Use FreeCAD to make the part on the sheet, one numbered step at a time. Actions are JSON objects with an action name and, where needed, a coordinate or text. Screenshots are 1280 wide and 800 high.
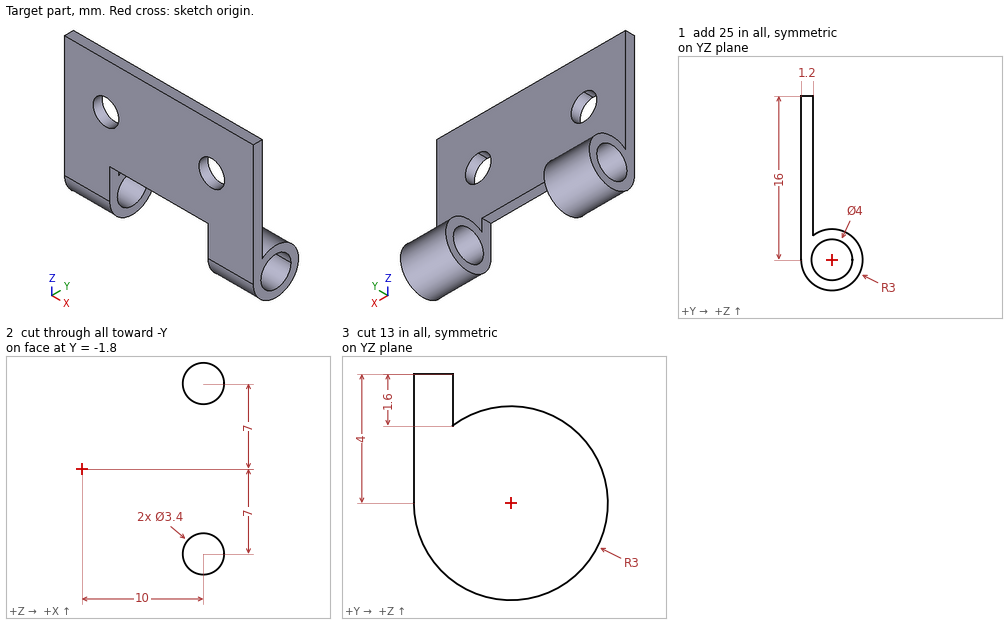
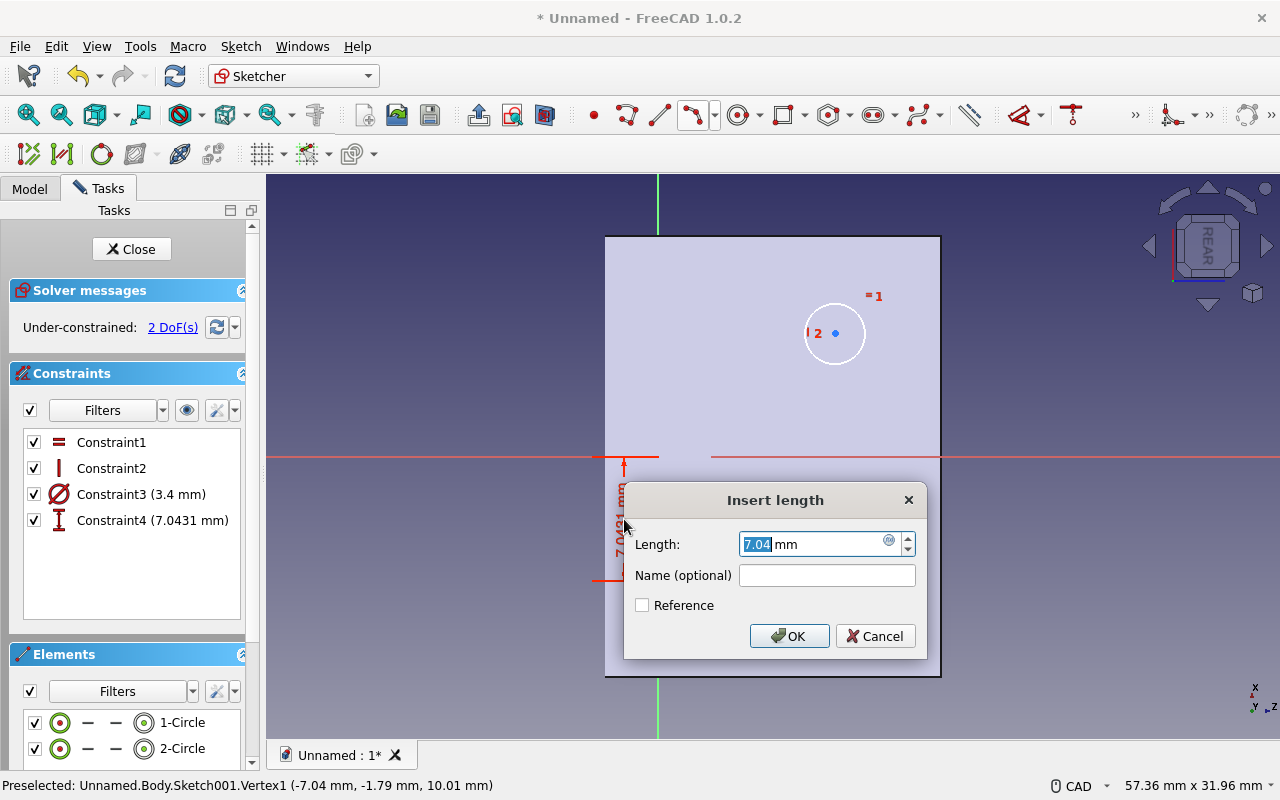
{"action": "type", "text": "7"}
{"action": "key", "text": "Return"}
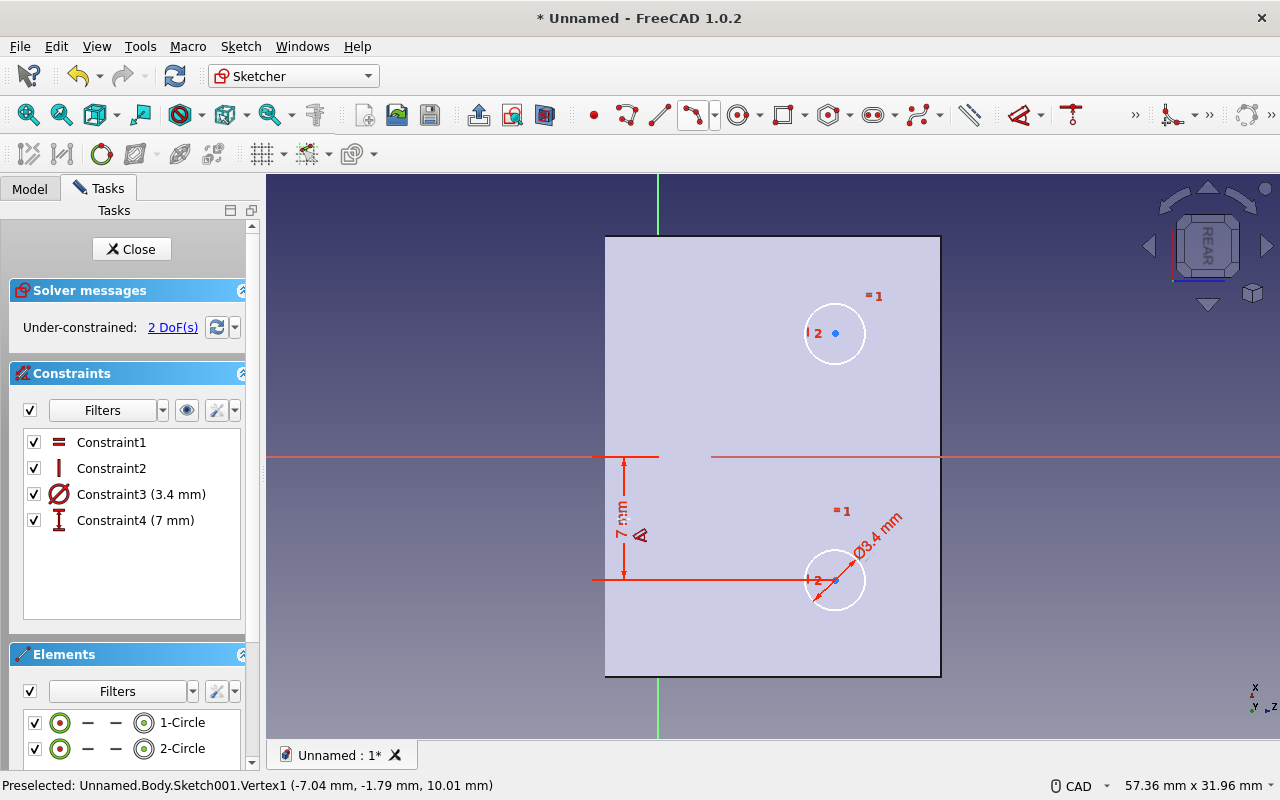
{"action": "left_click", "coordinate": [835, 334]}
{"action": "left_click", "coordinate": [624, 395]}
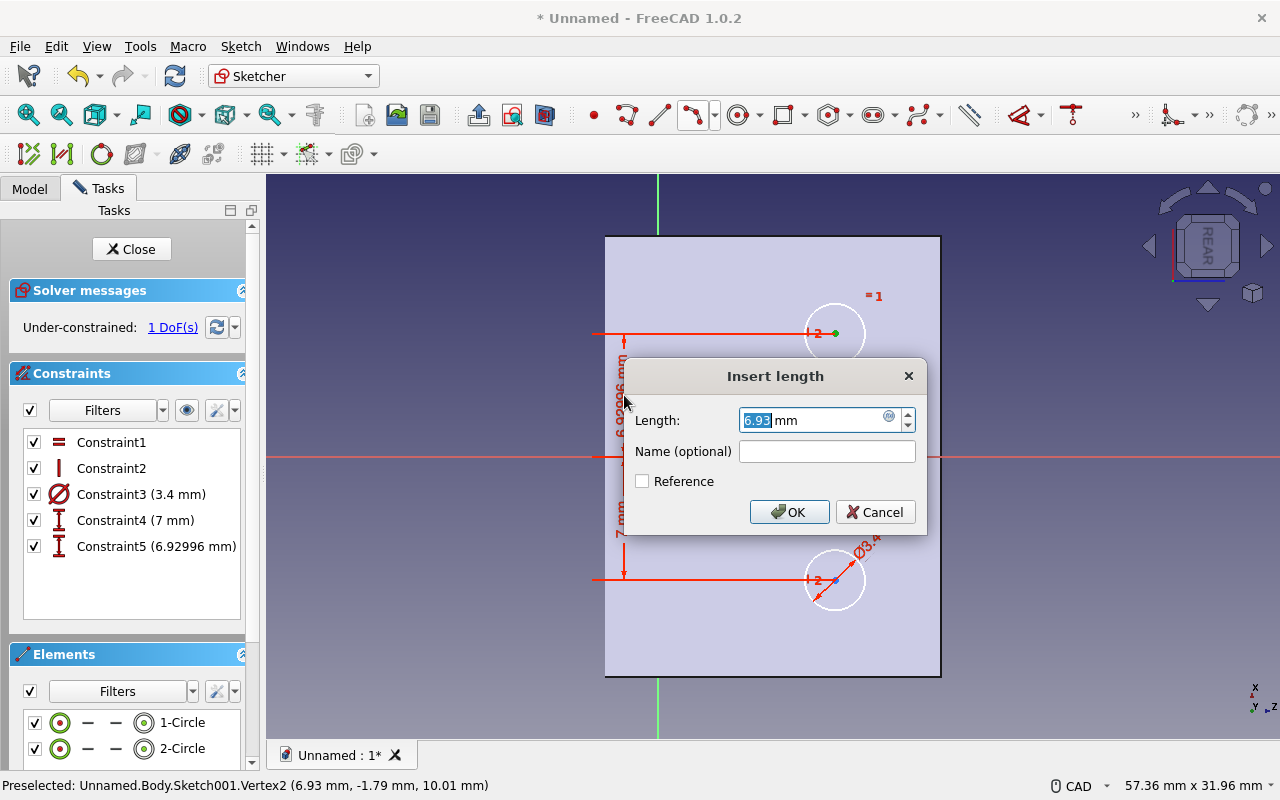
{"action": "type", "text": "7"}
{"action": "key", "text": "Return"}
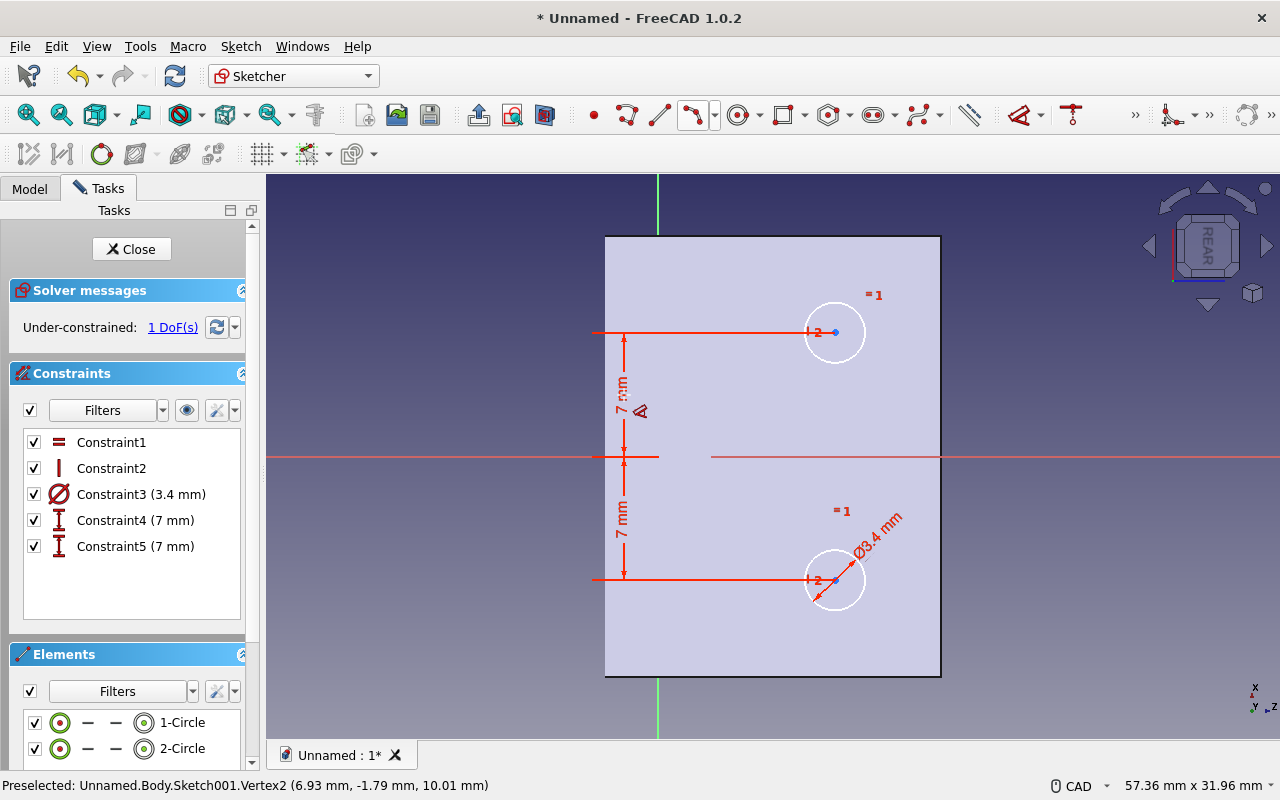
{"action": "left_click", "coordinate": [835, 580]}
{"action": "left_click", "coordinate": [747, 614]}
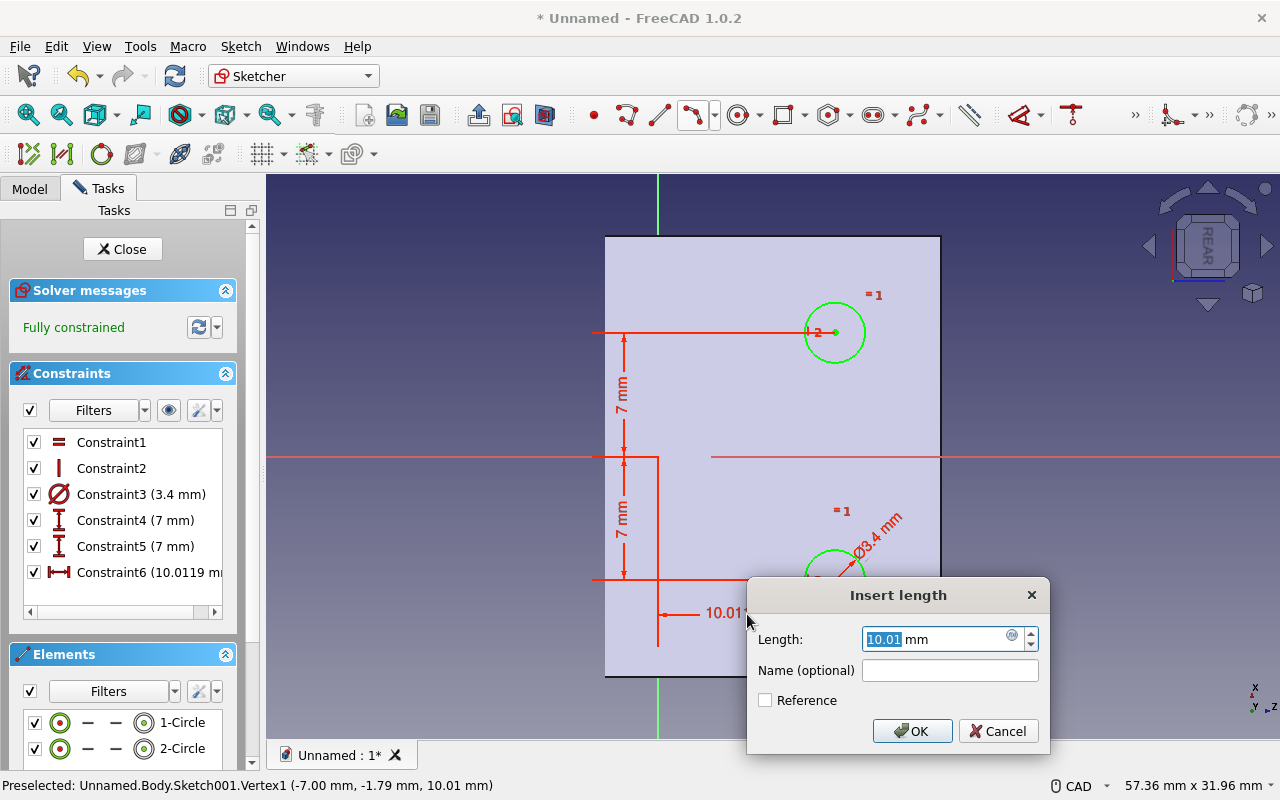
{"action": "type", "text": "10"}
{"action": "key", "text": "Return"}
{"action": "key", "text": "Escape"}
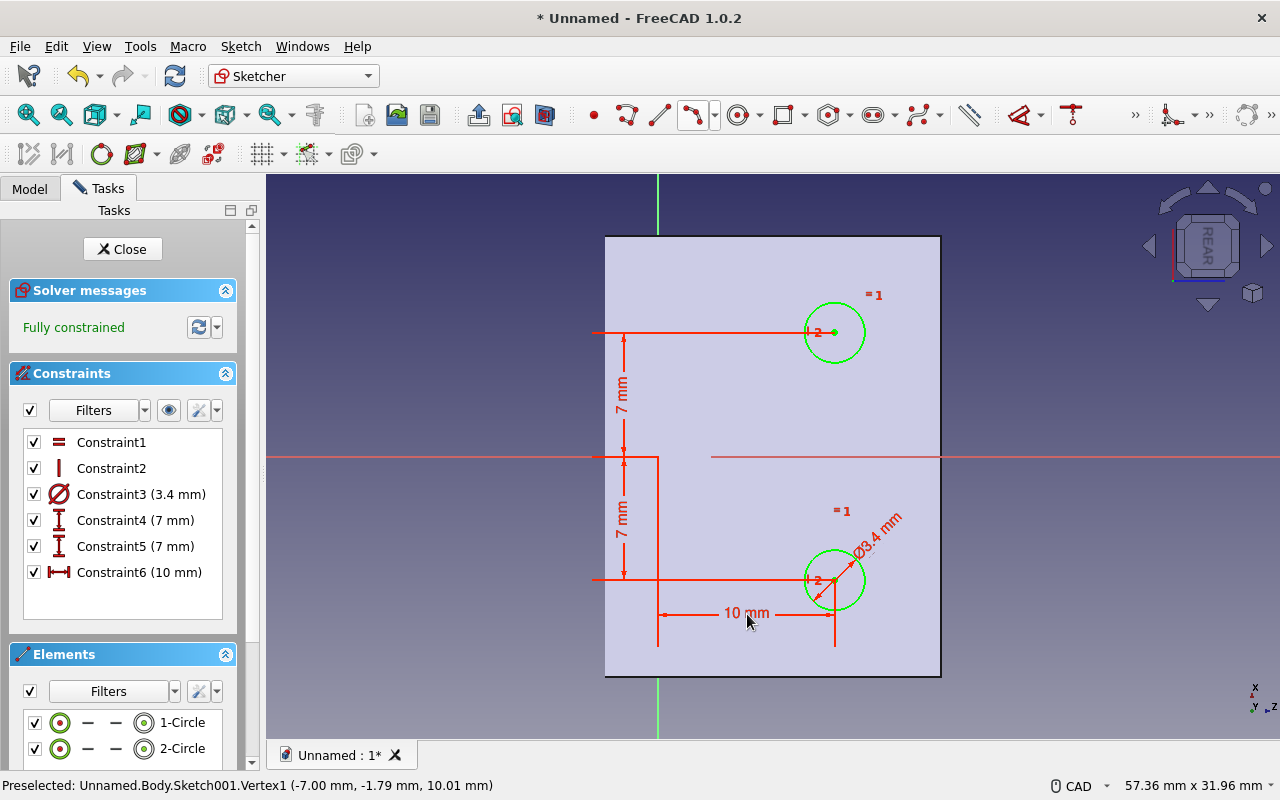
{"action": "left_click", "coordinate": [123, 249]}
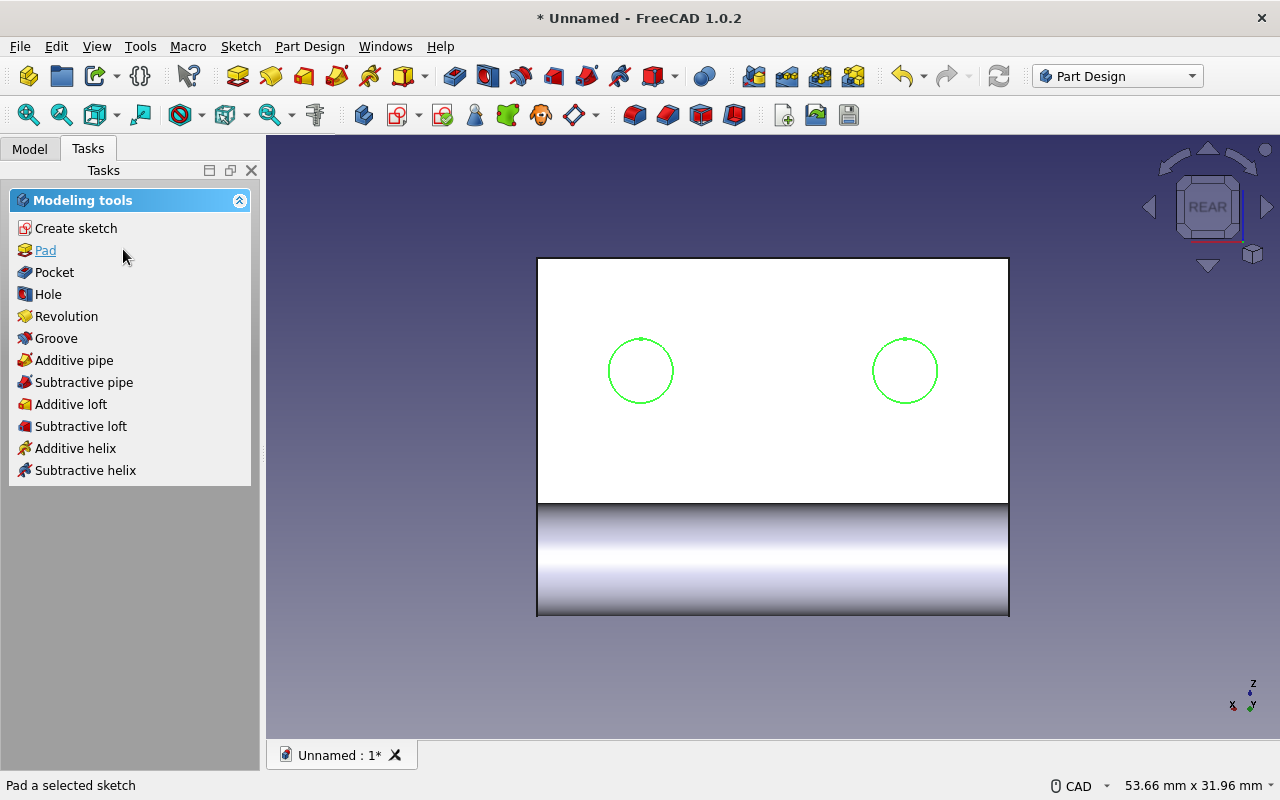
{"action": "left_click", "coordinate": [455, 76]}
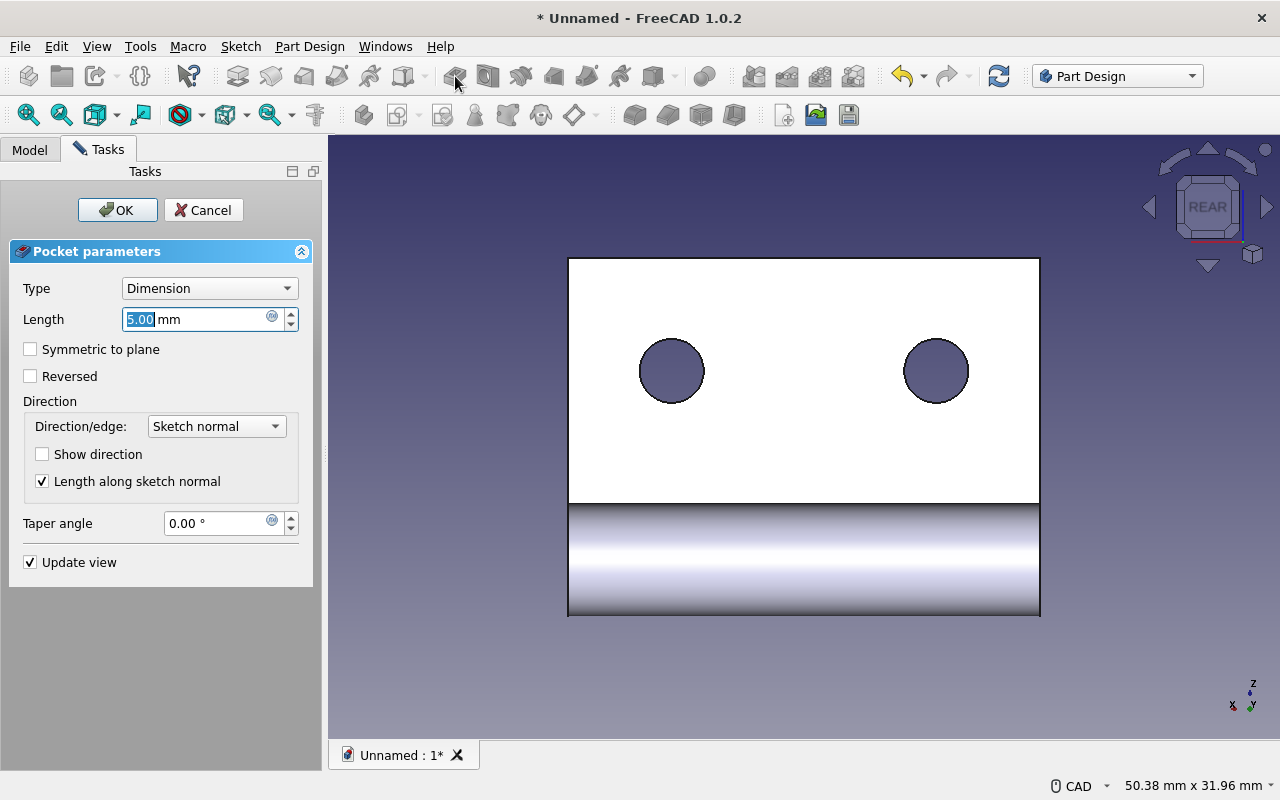
{"action": "left_click", "coordinate": [210, 288]}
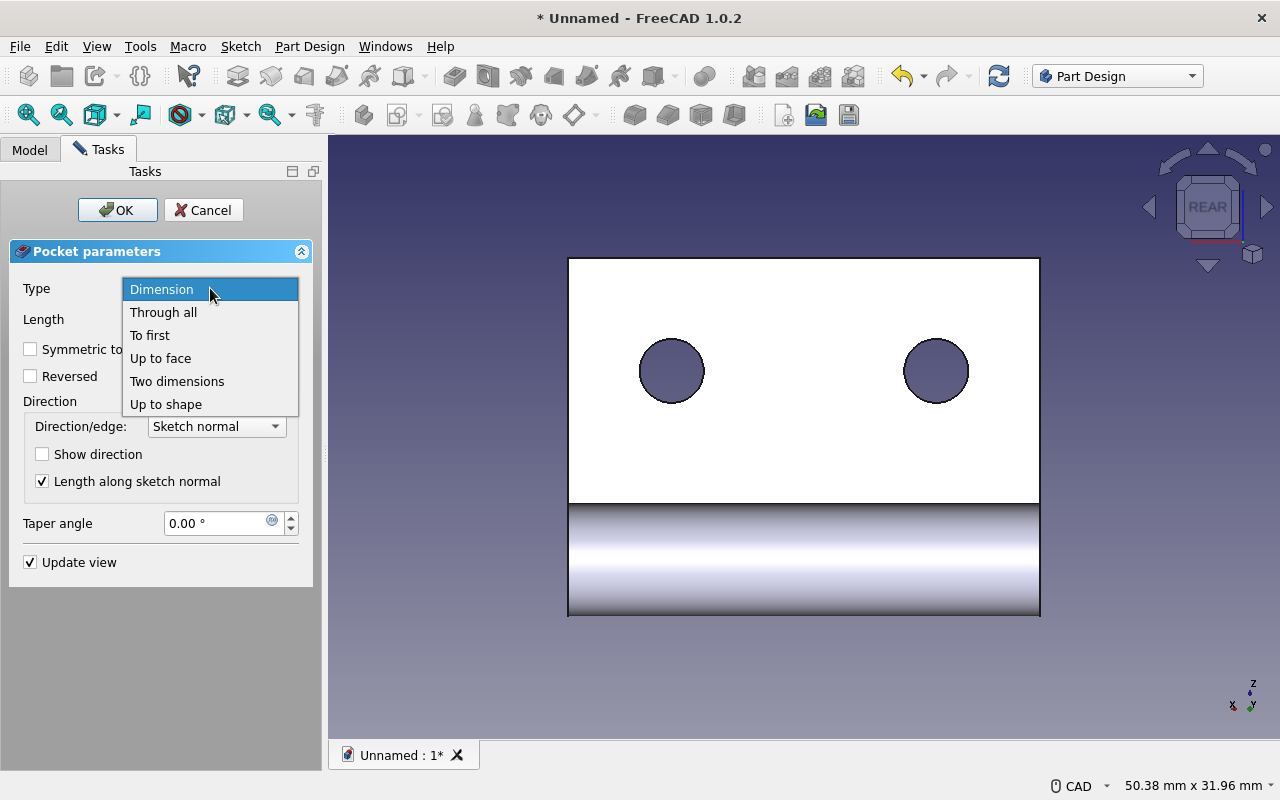
{"action": "left_click", "coordinate": [208, 312]}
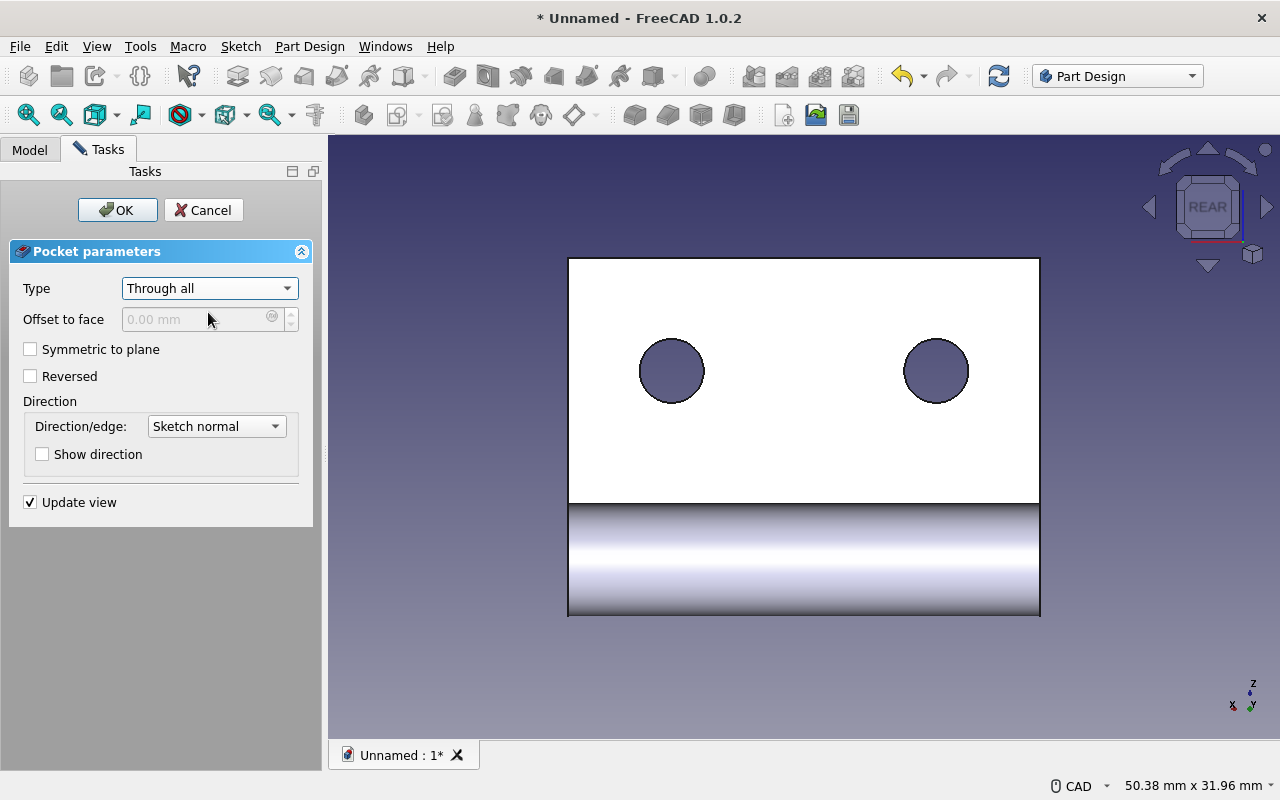
{"action": "left_click", "coordinate": [118, 210]}